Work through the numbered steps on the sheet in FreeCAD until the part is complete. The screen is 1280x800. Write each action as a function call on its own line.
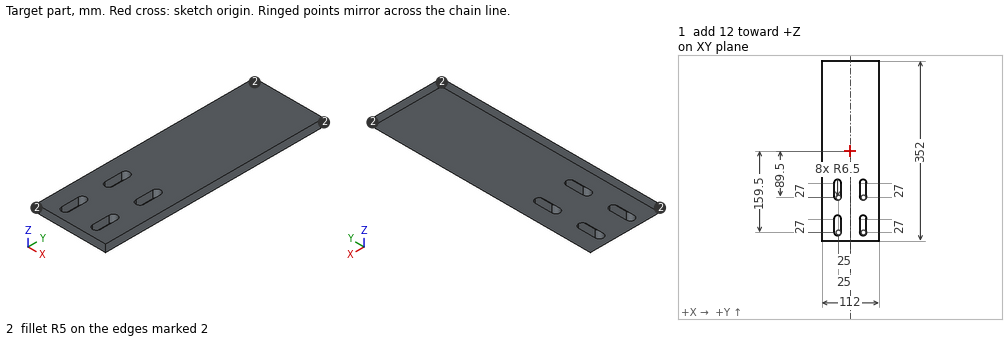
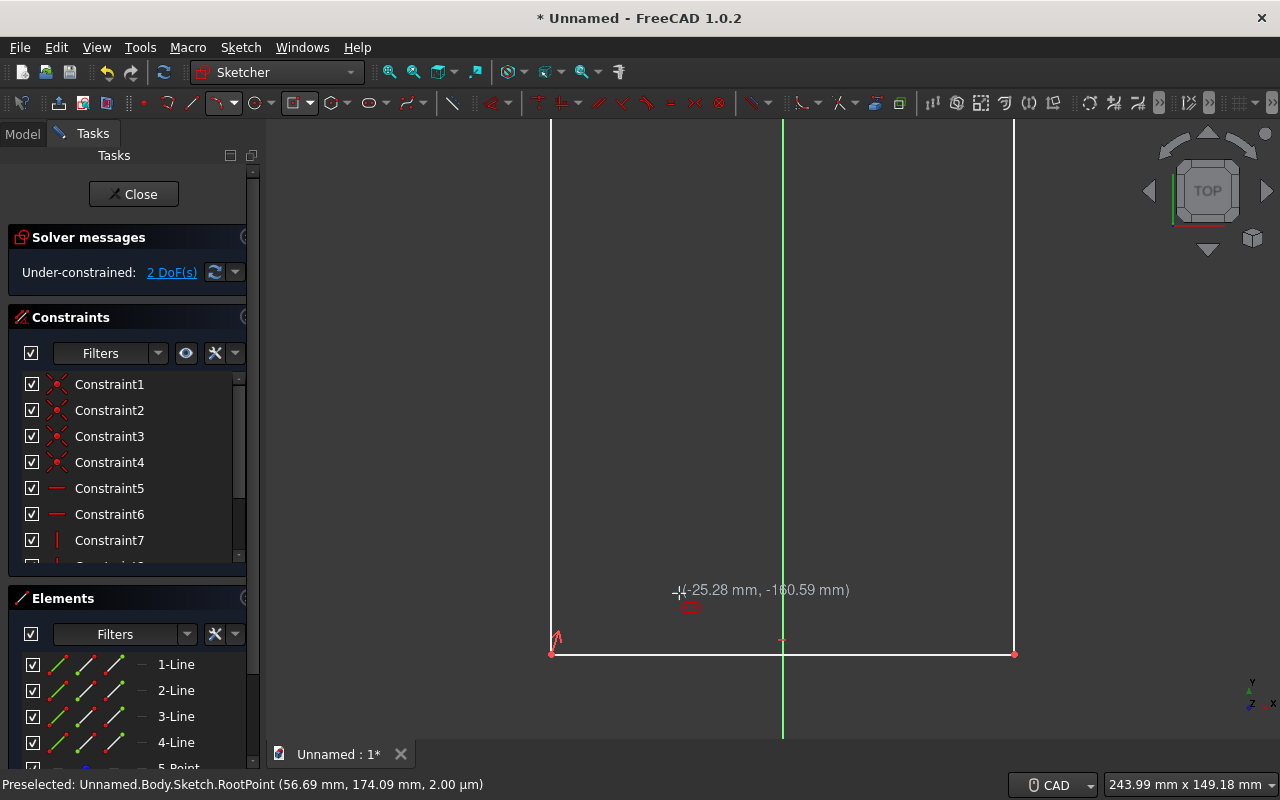
scroll(679, 593, down, 7)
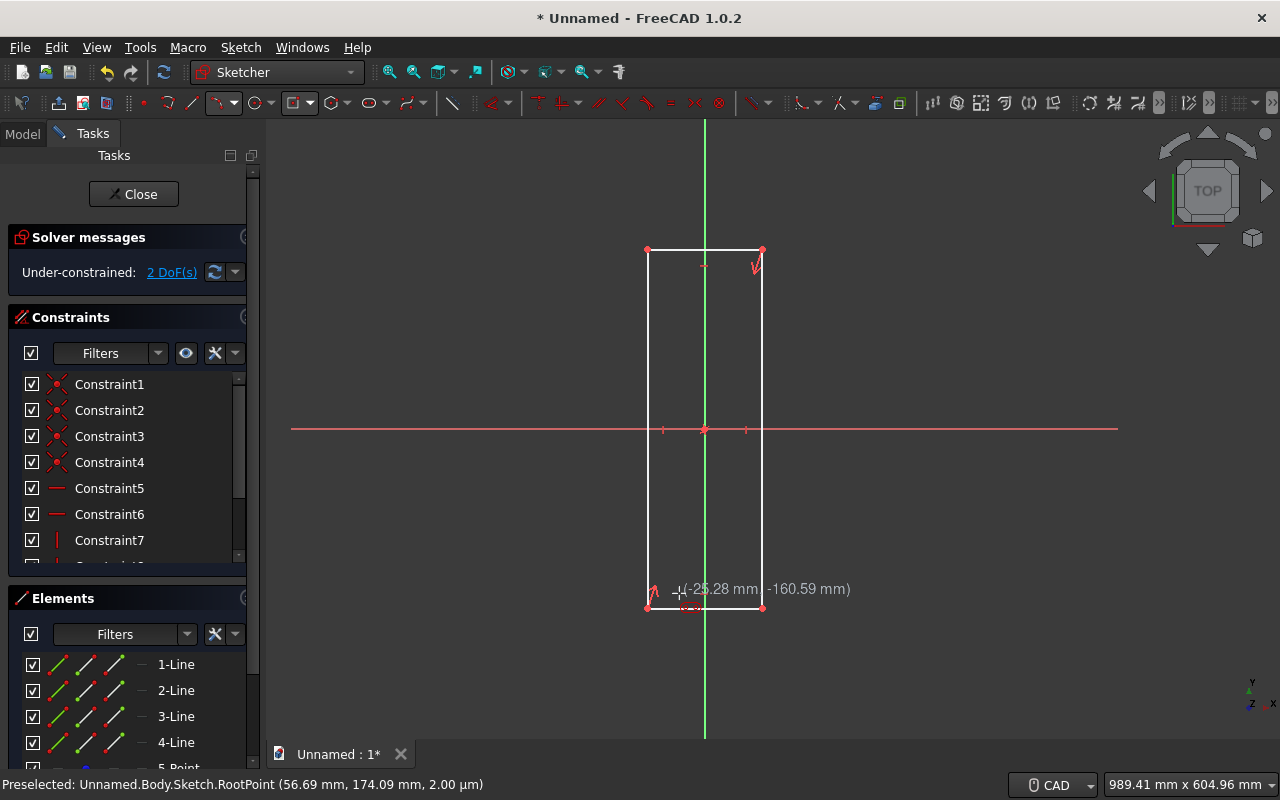
click(679, 593)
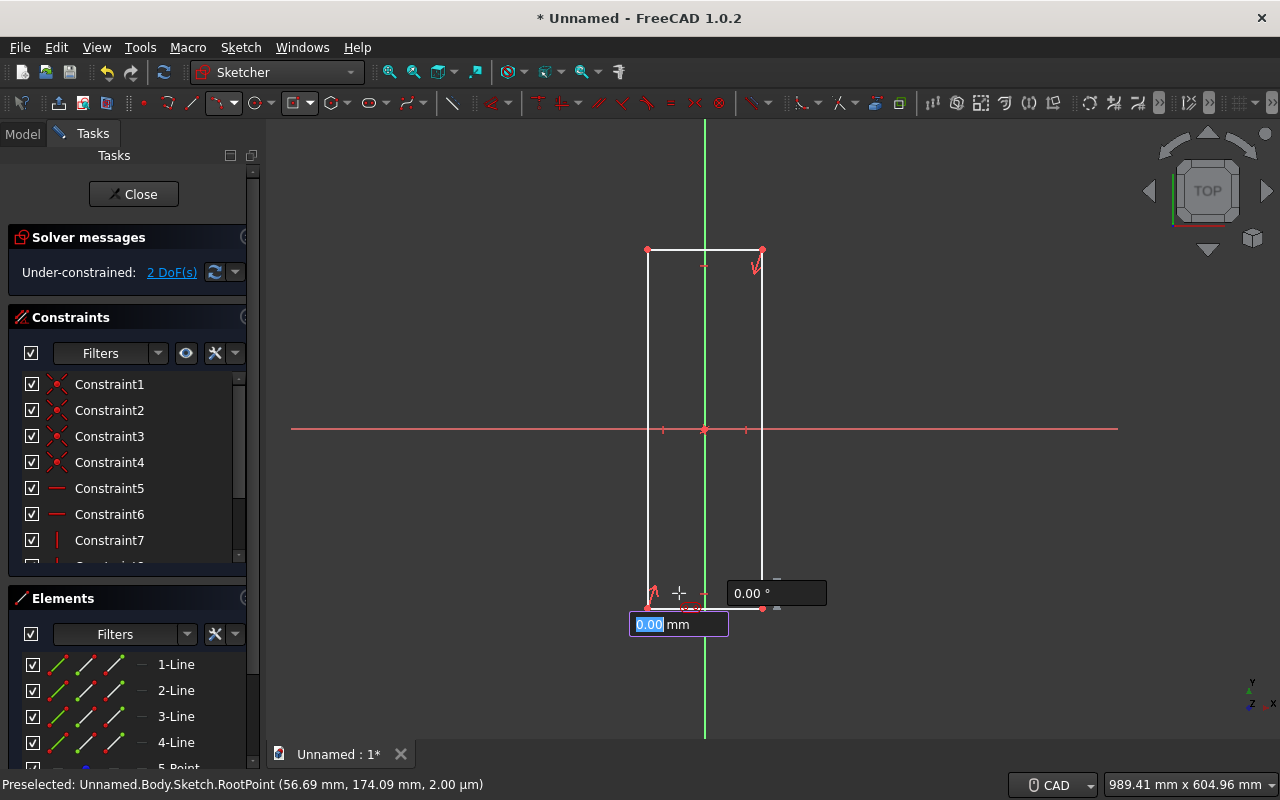
click(679, 565)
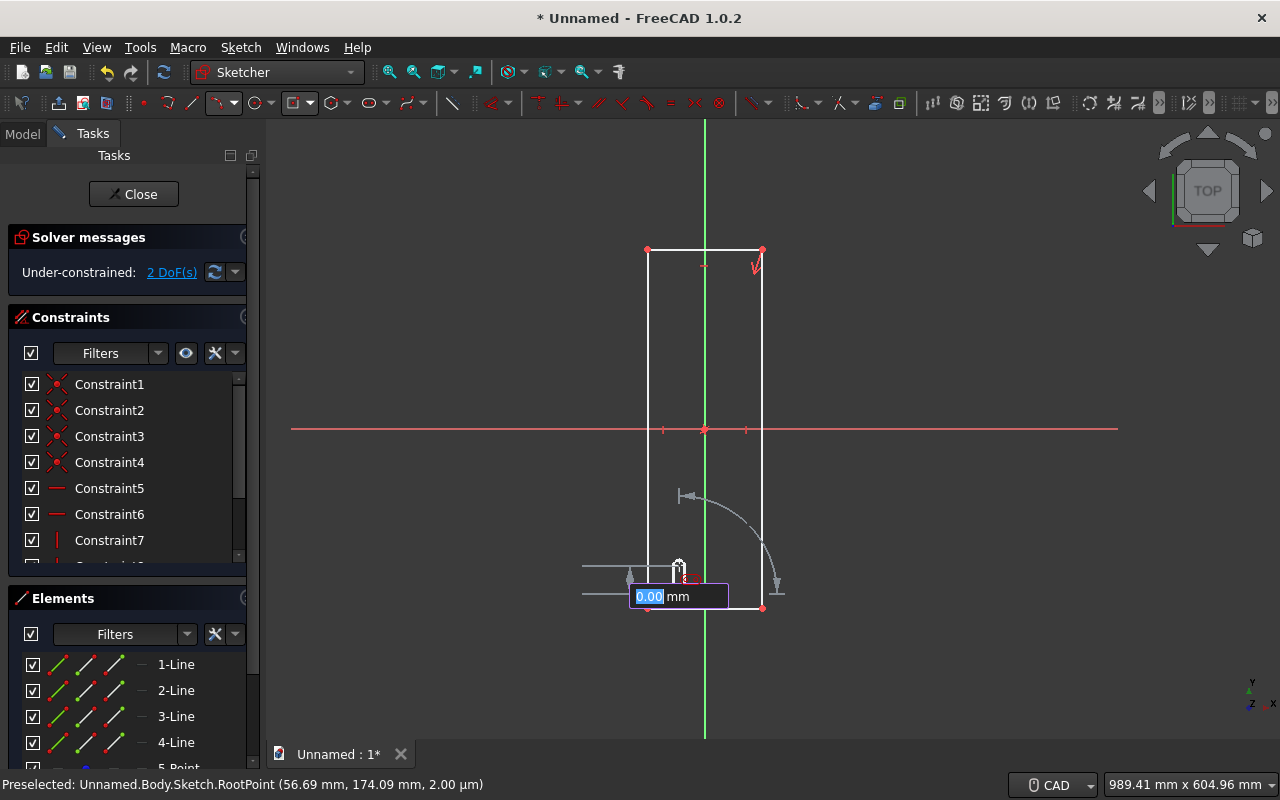
scroll(673, 579, up, 5)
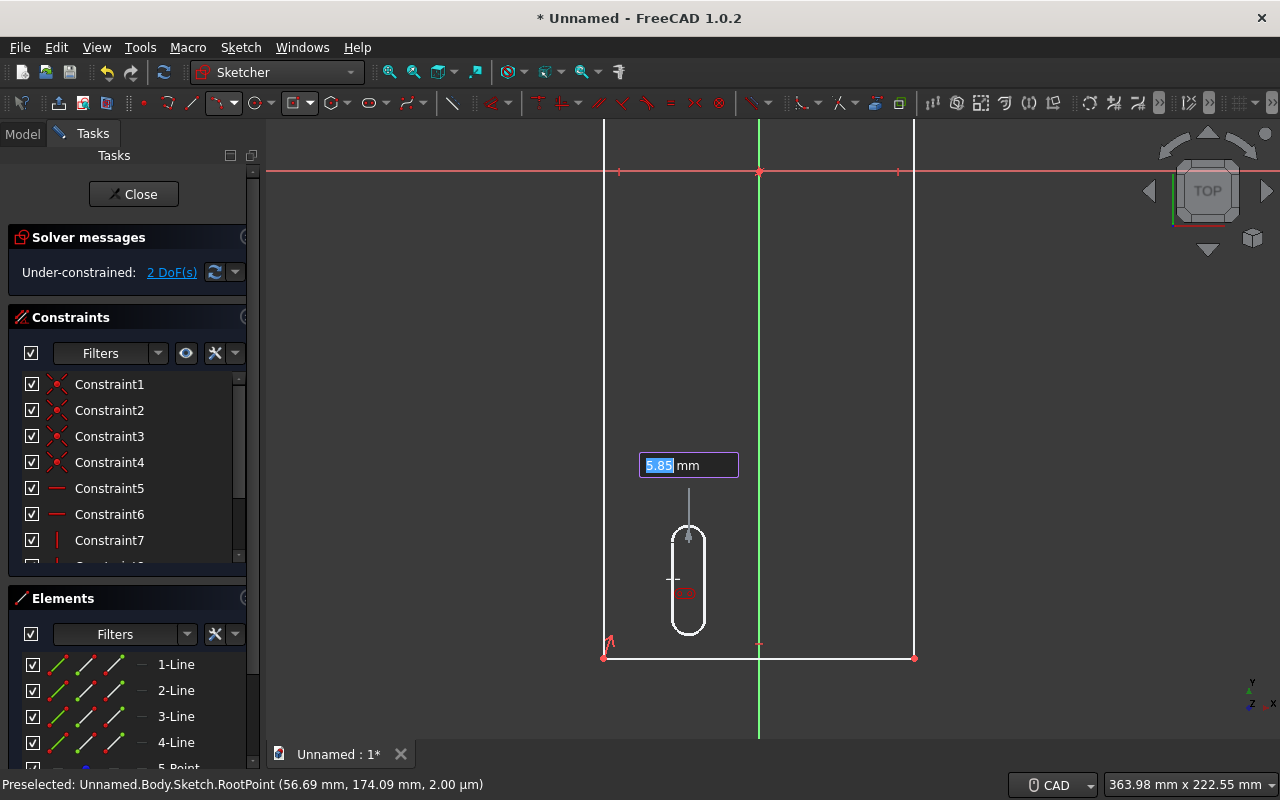
click(671, 578)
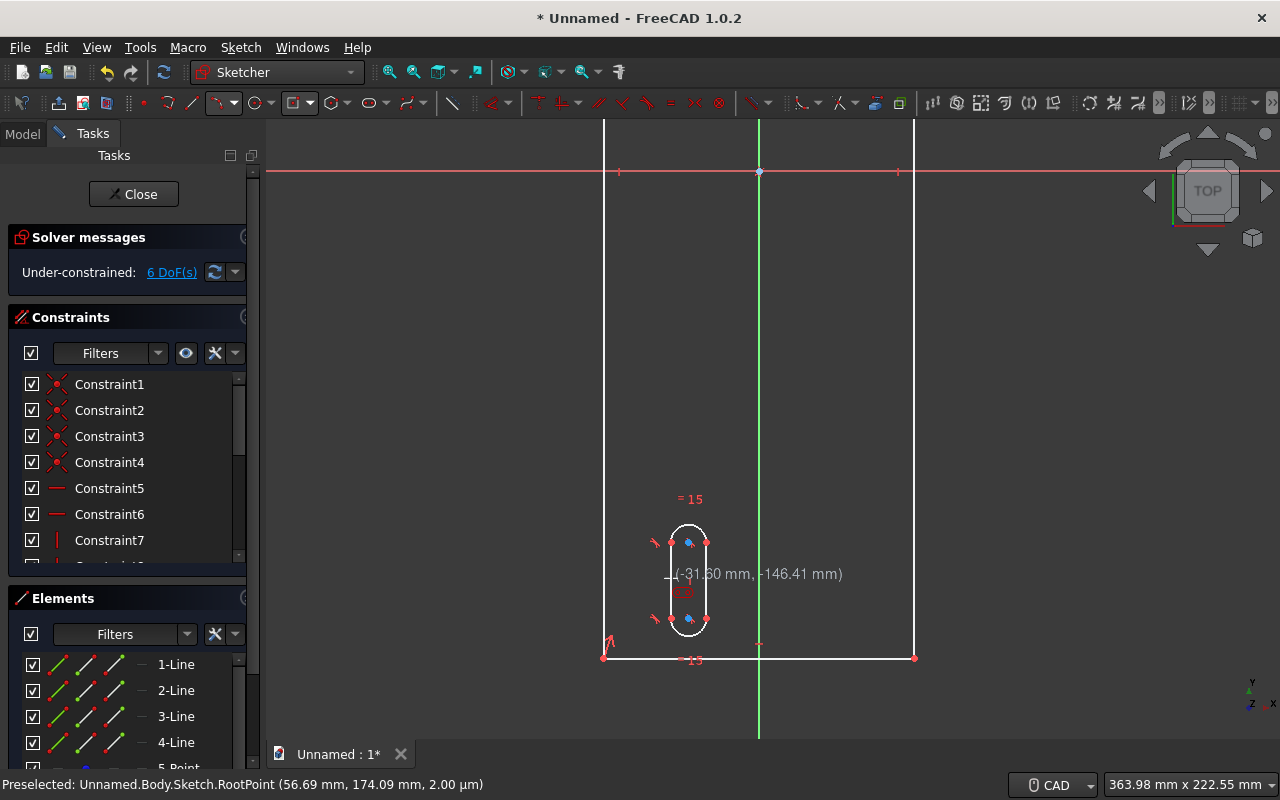
scroll(829, 615, up, 2)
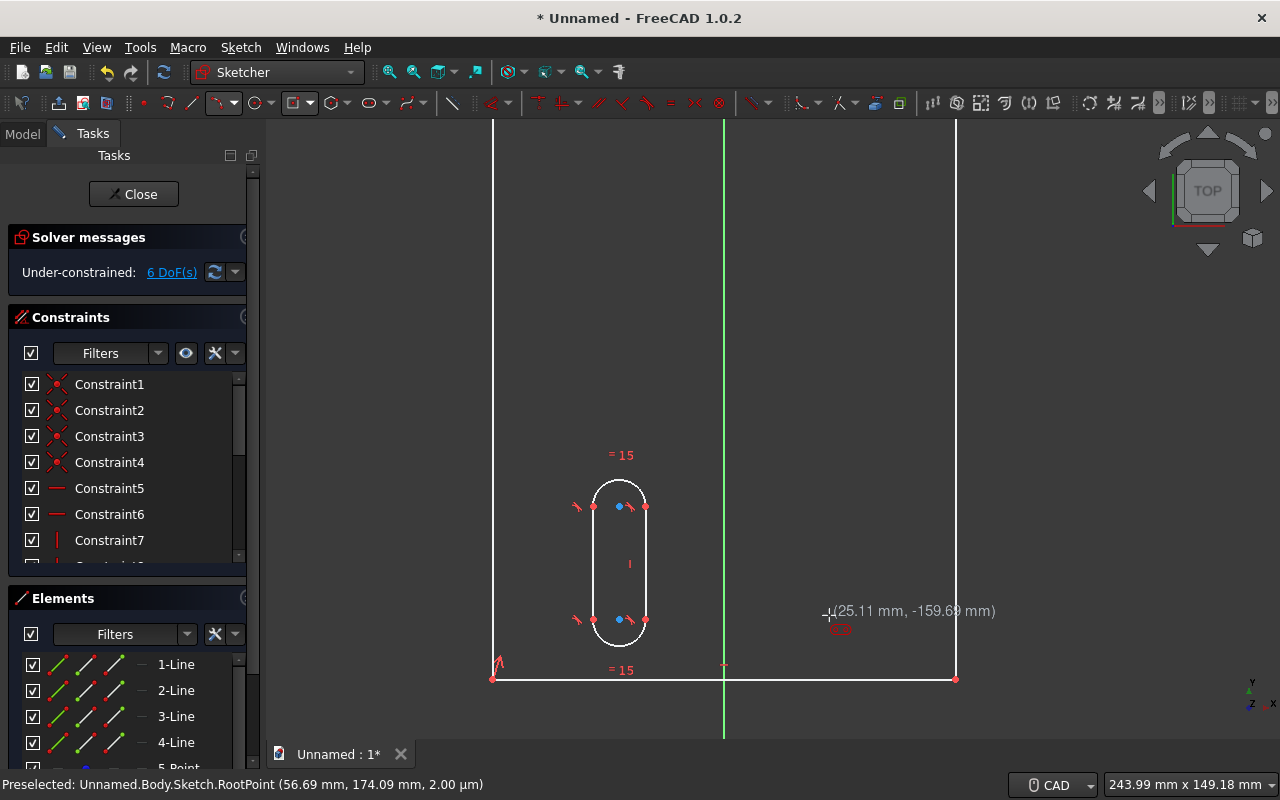
scroll(698, 585, down, 7)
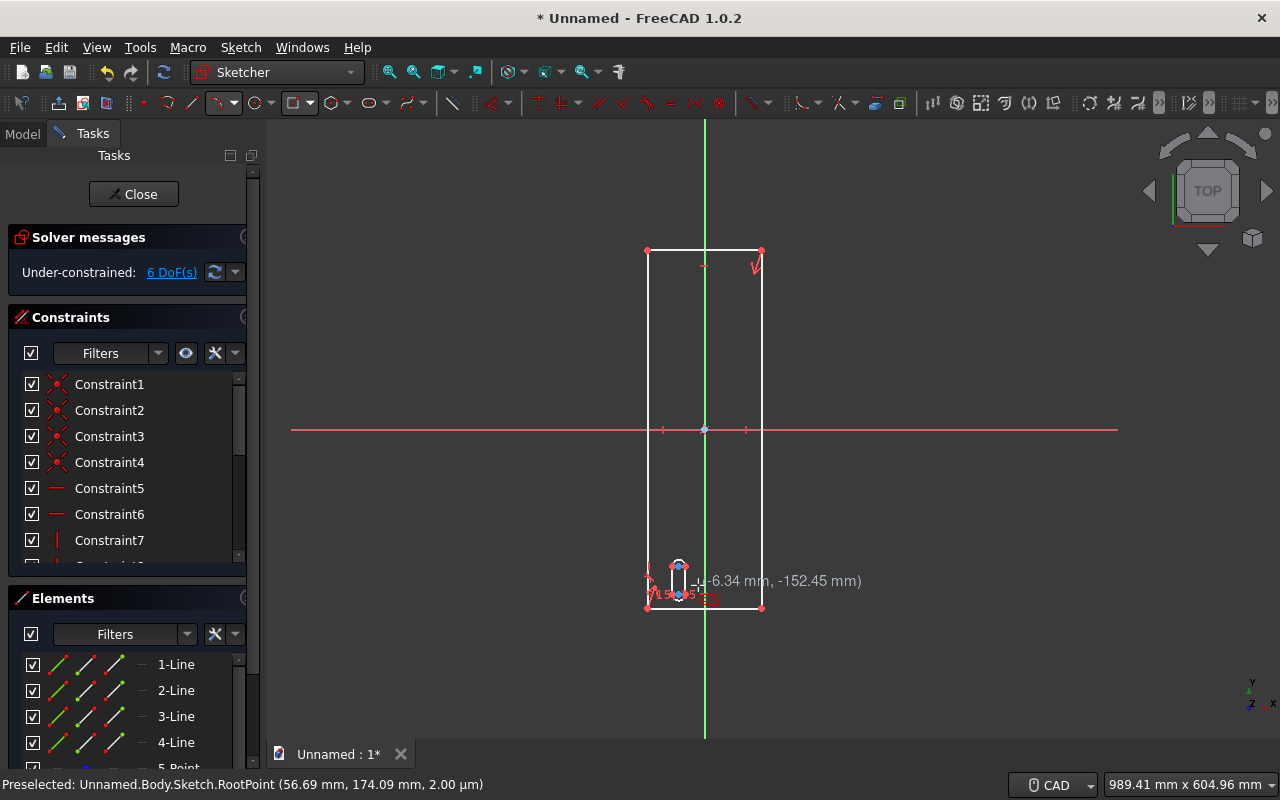
click(730, 593)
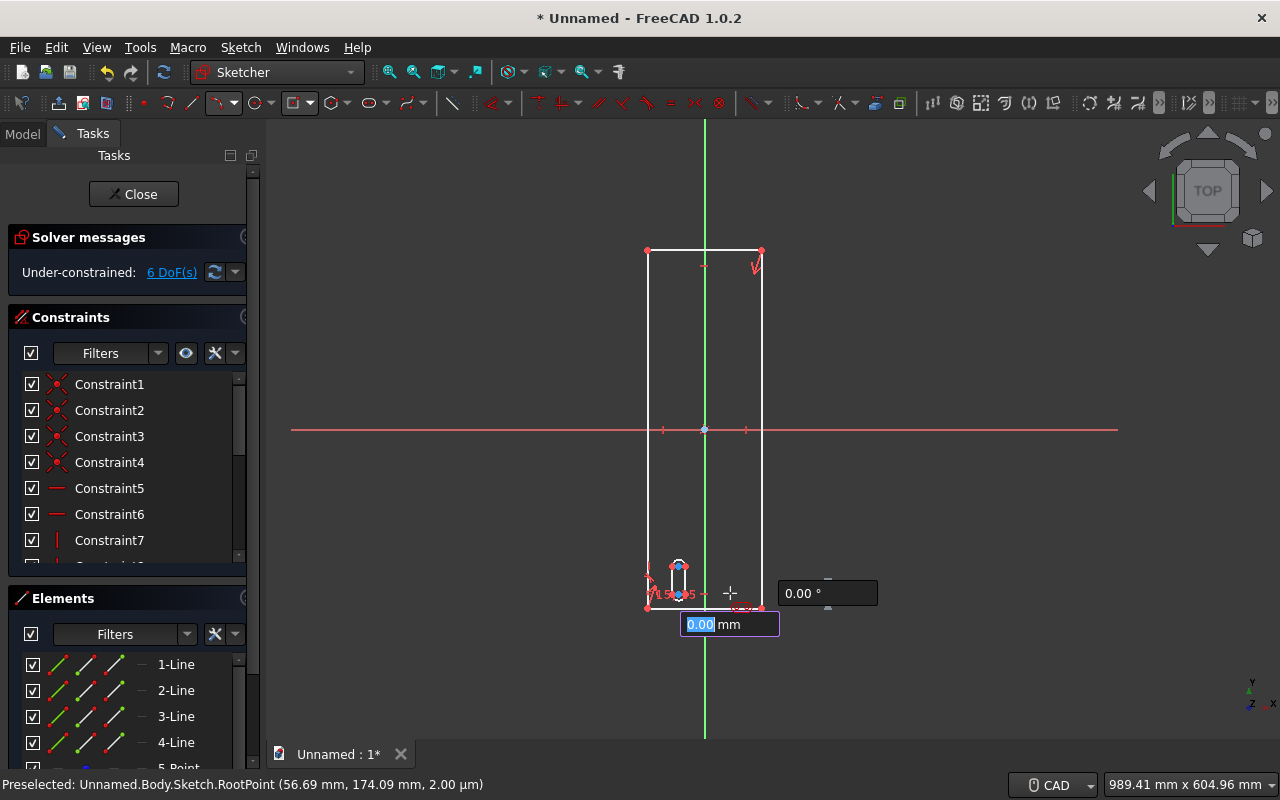
click(730, 565)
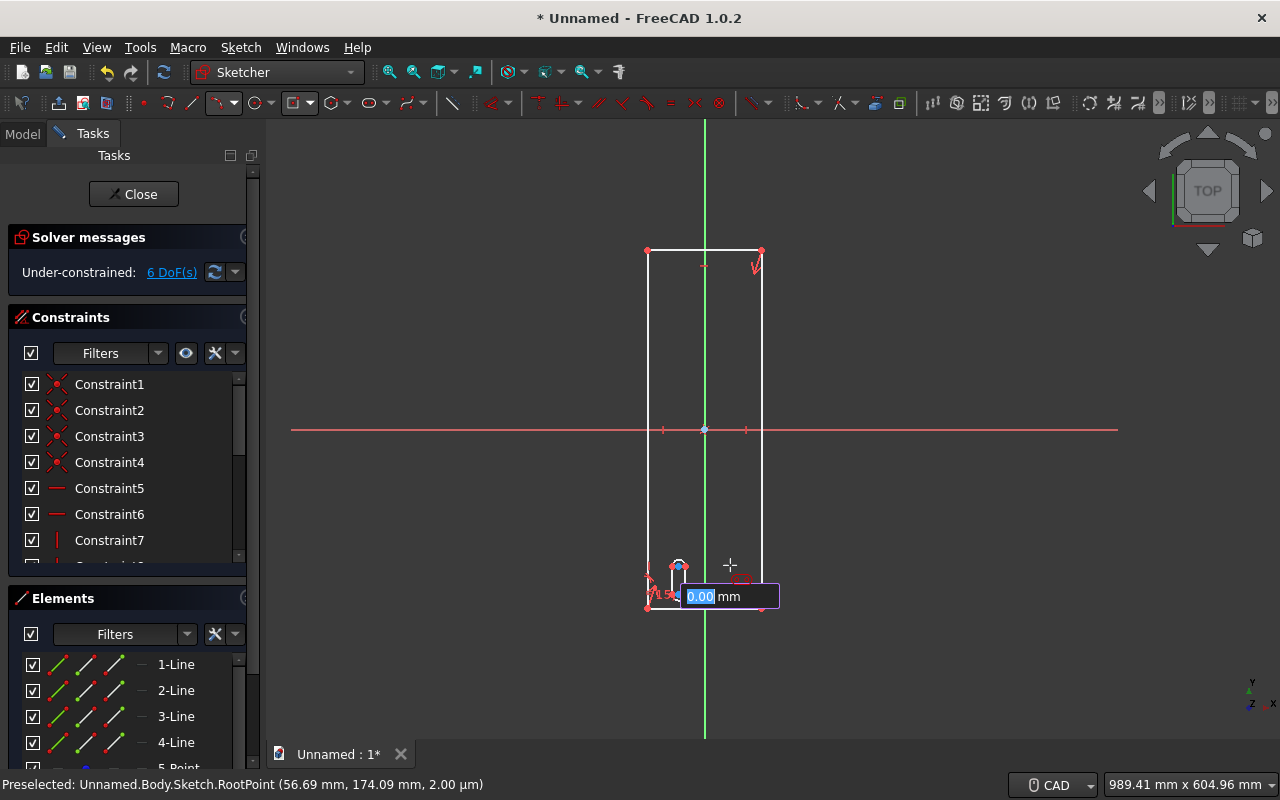
scroll(724, 579, up, 5)